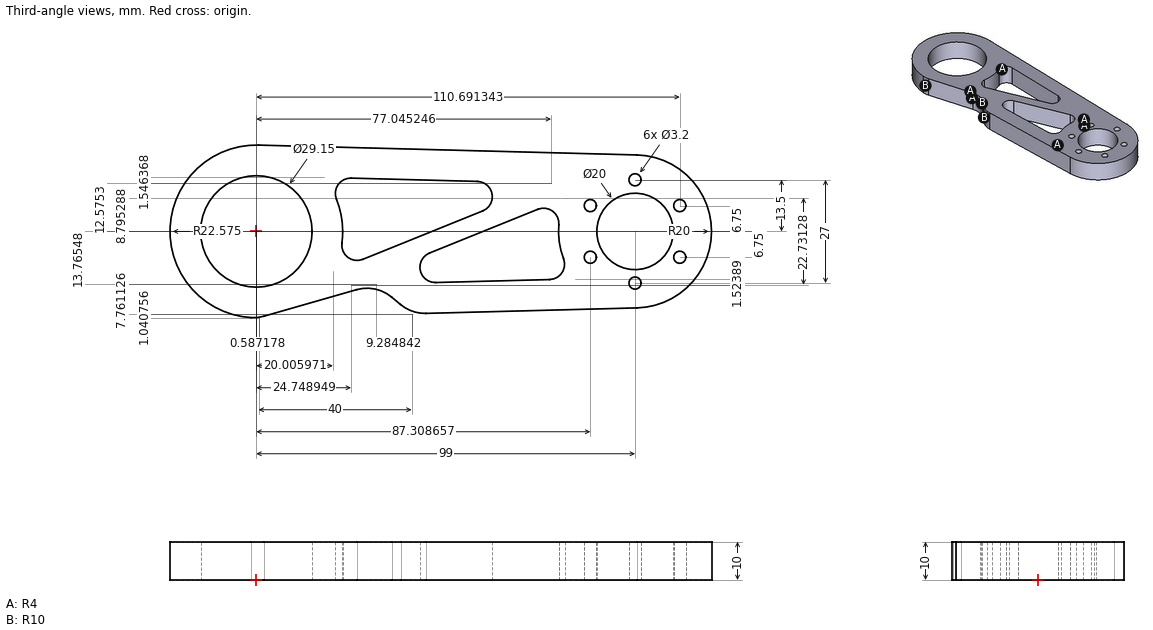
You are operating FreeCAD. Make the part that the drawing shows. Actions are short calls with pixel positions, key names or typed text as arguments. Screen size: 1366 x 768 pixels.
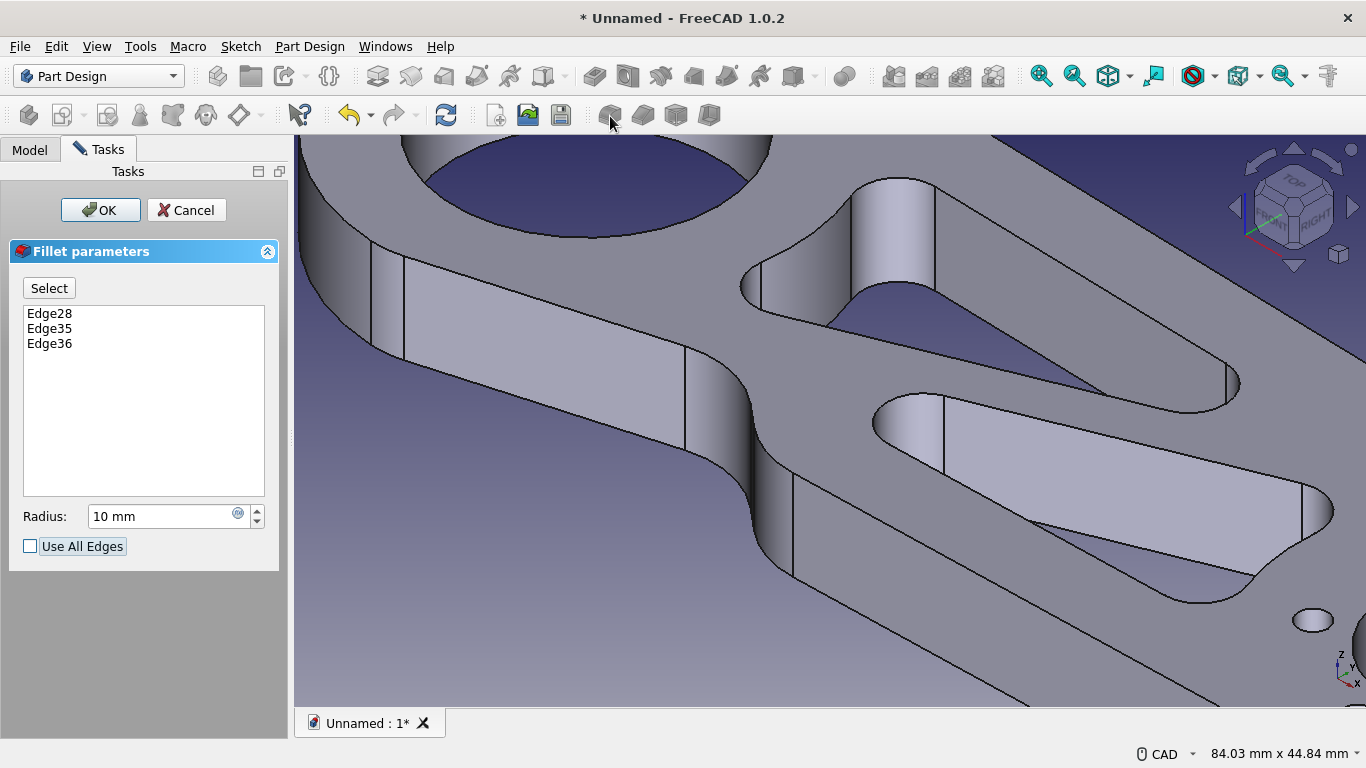
click(101, 210)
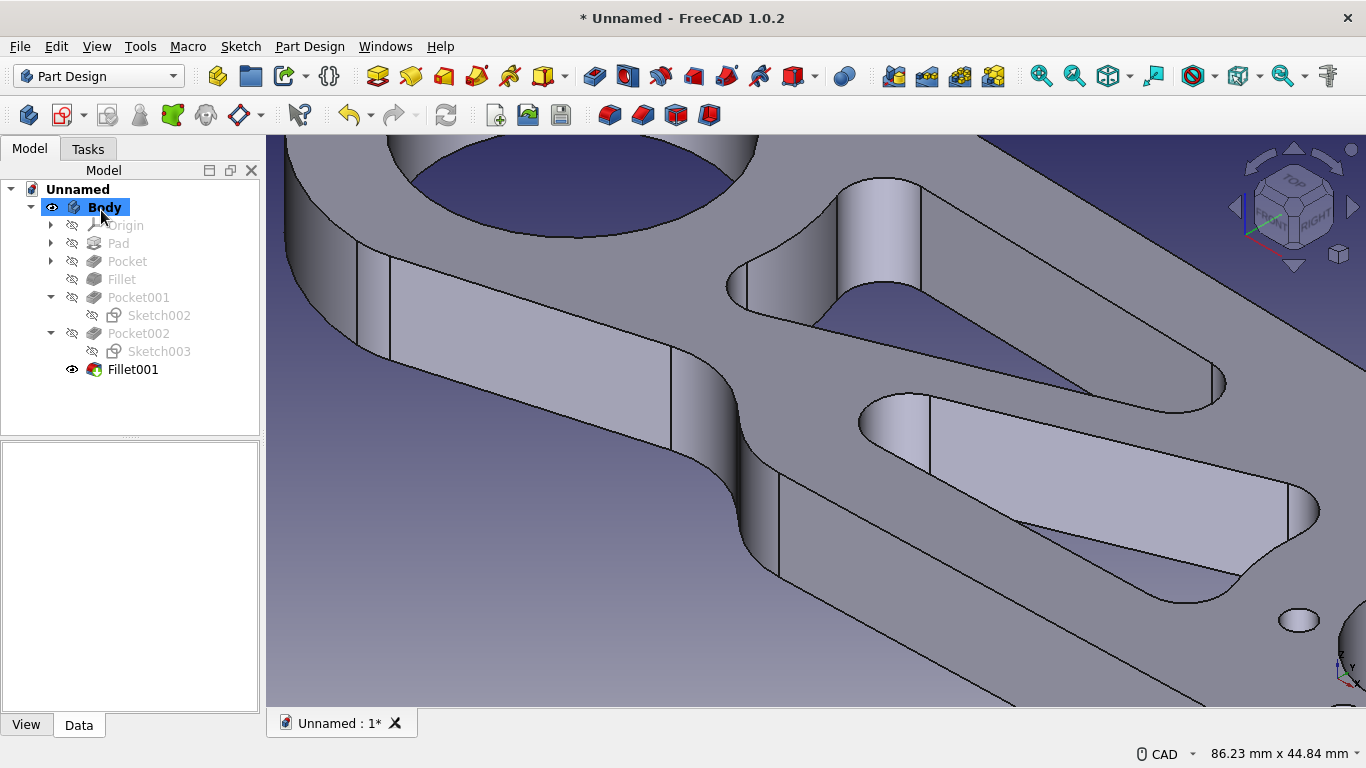
key(v)
key(f)